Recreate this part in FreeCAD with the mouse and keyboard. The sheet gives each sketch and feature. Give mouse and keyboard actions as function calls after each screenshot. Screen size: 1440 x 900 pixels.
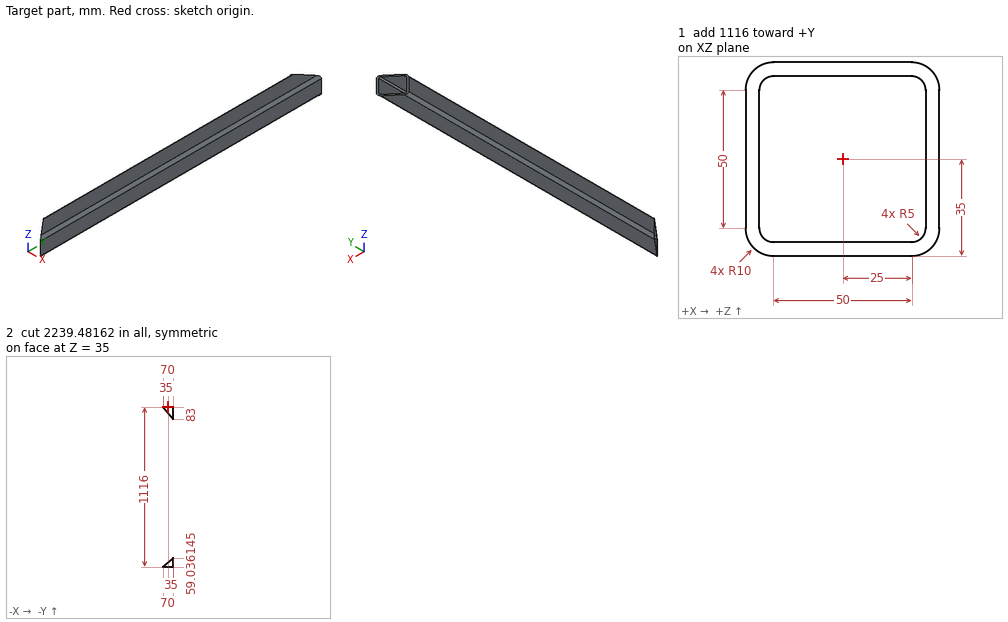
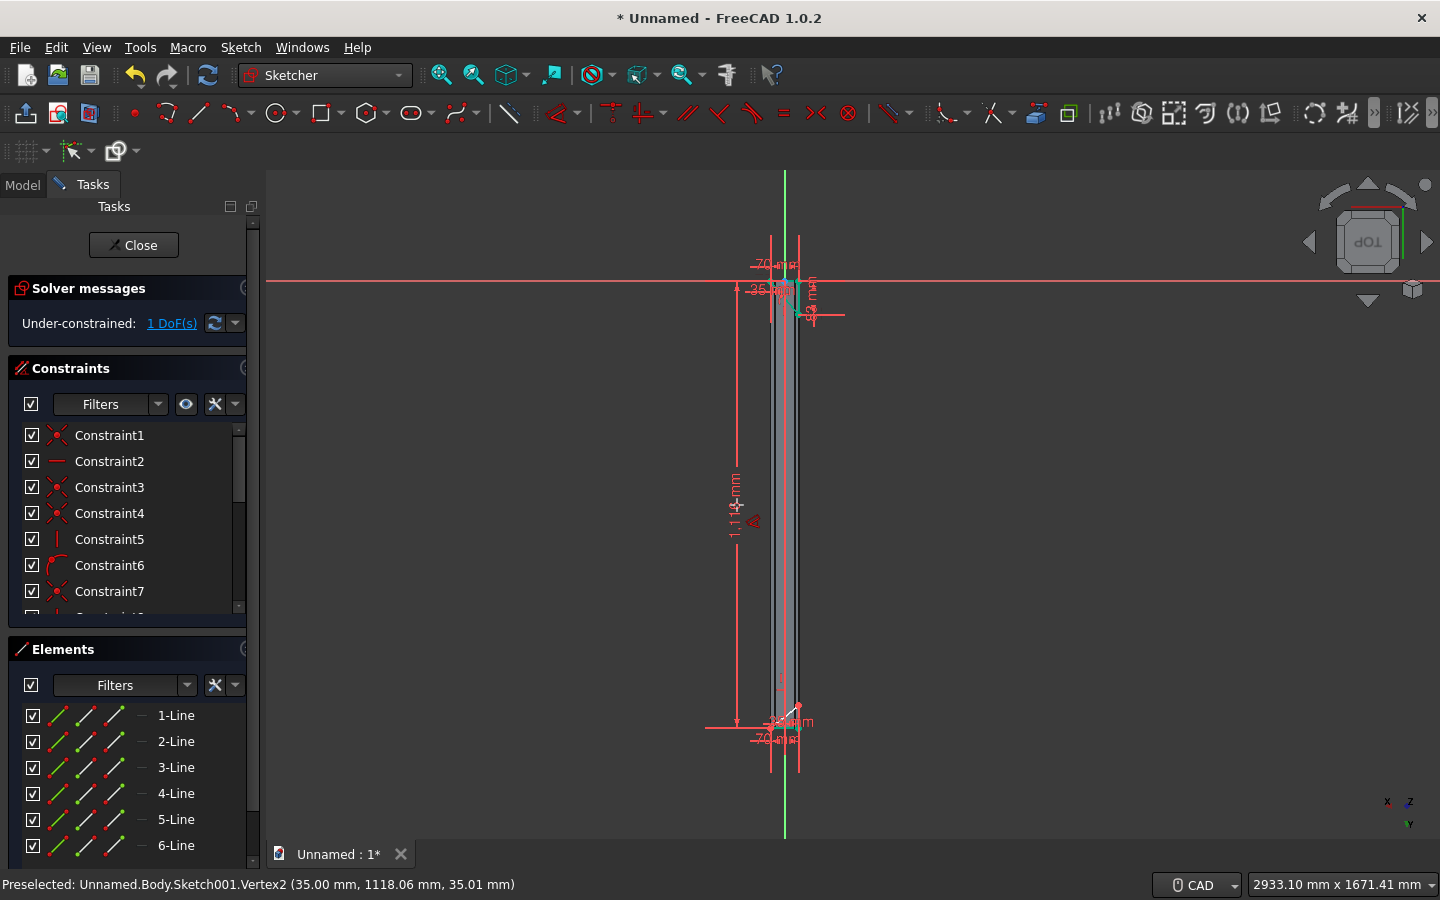
scroll(799, 719, up, 3)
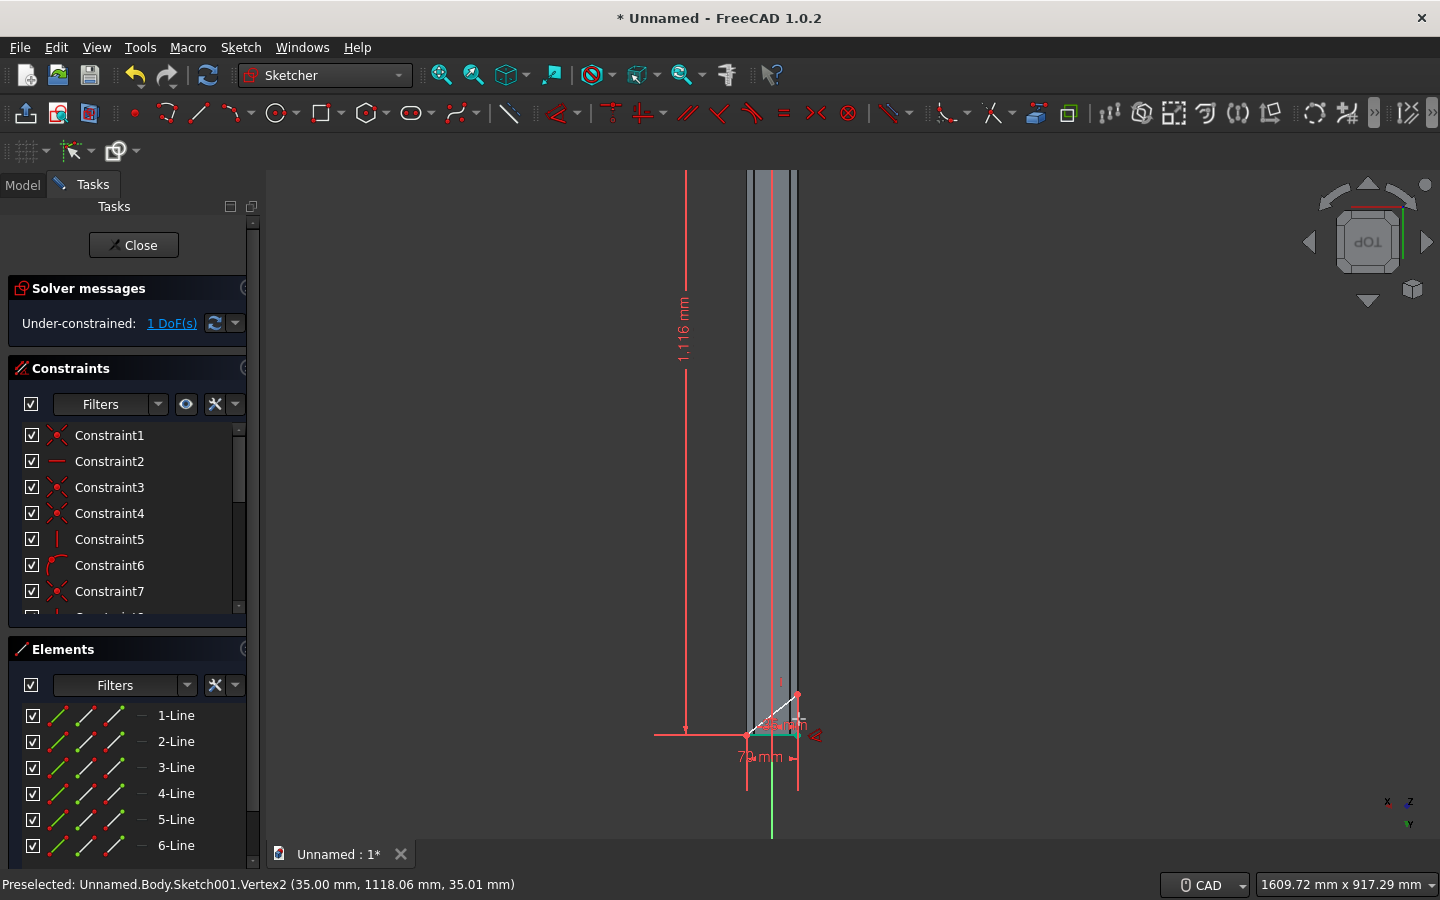
click(798, 719)
click(832, 706)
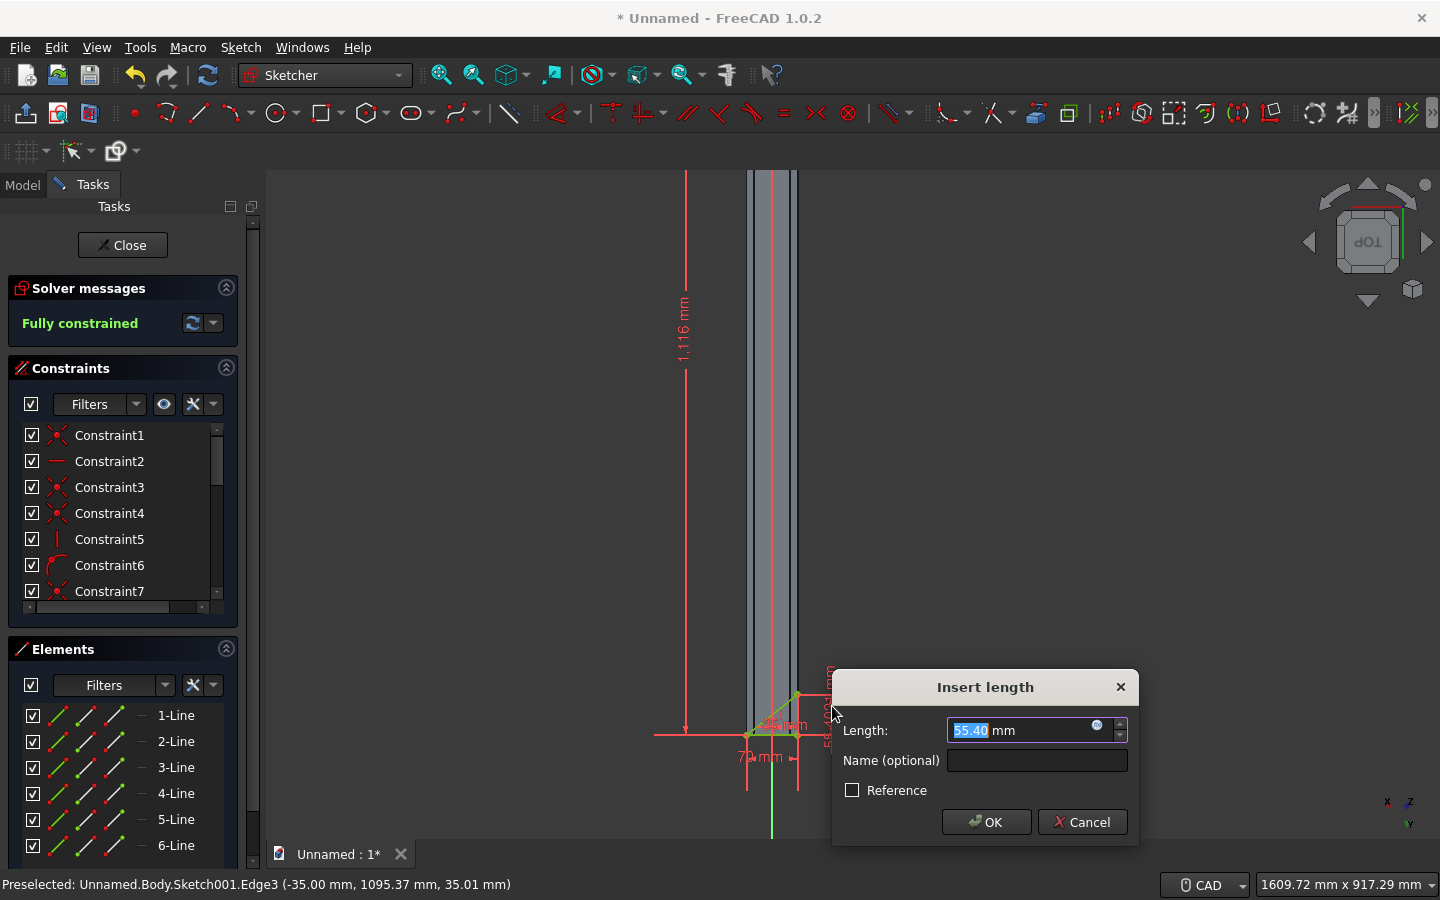
text(59.036145)
key(Return)
key(Escape)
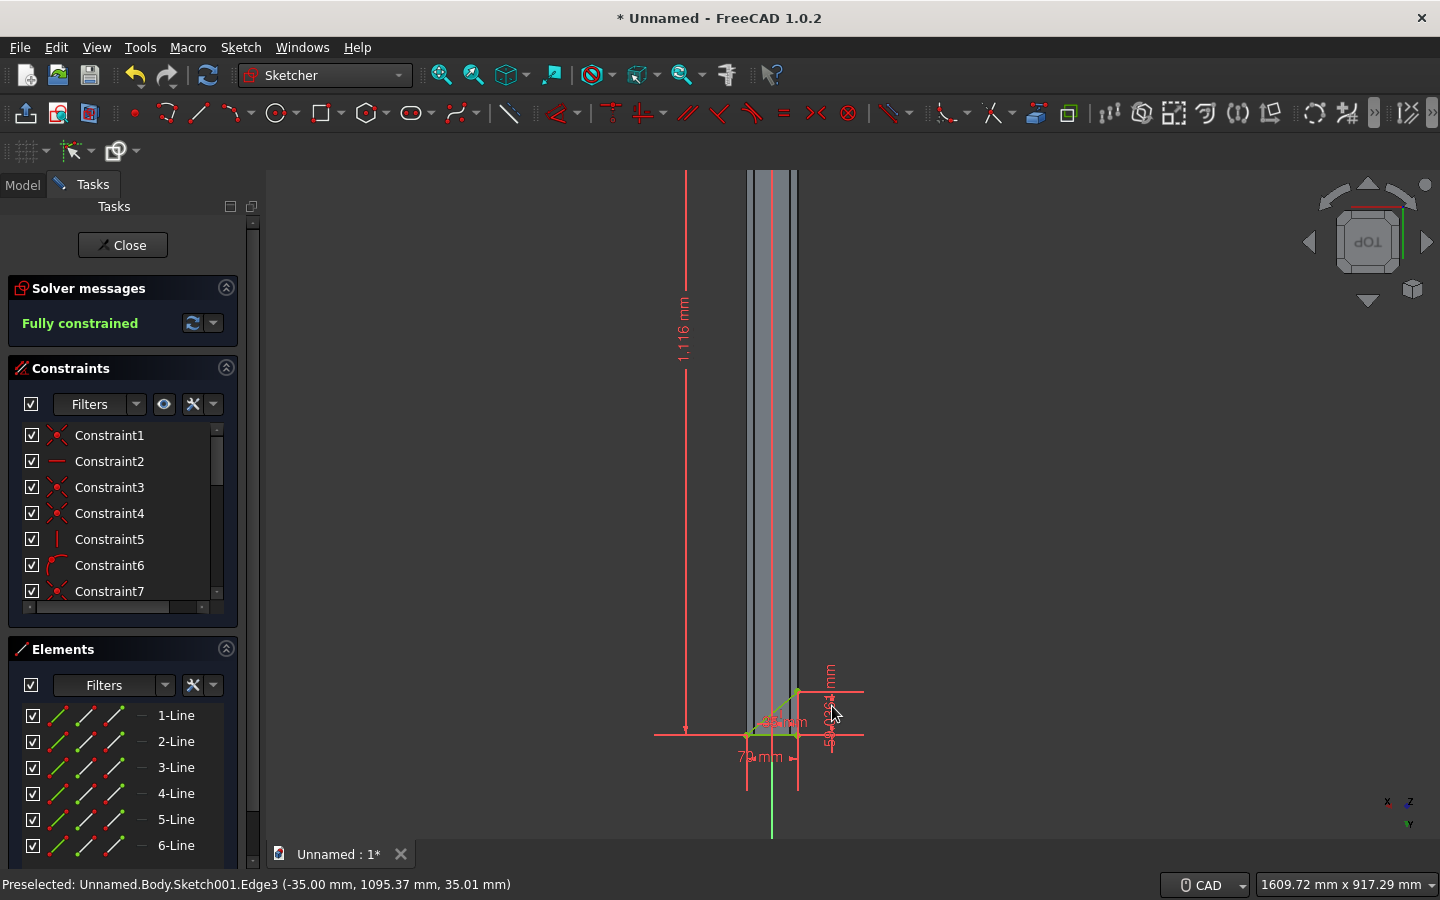
click(123, 245)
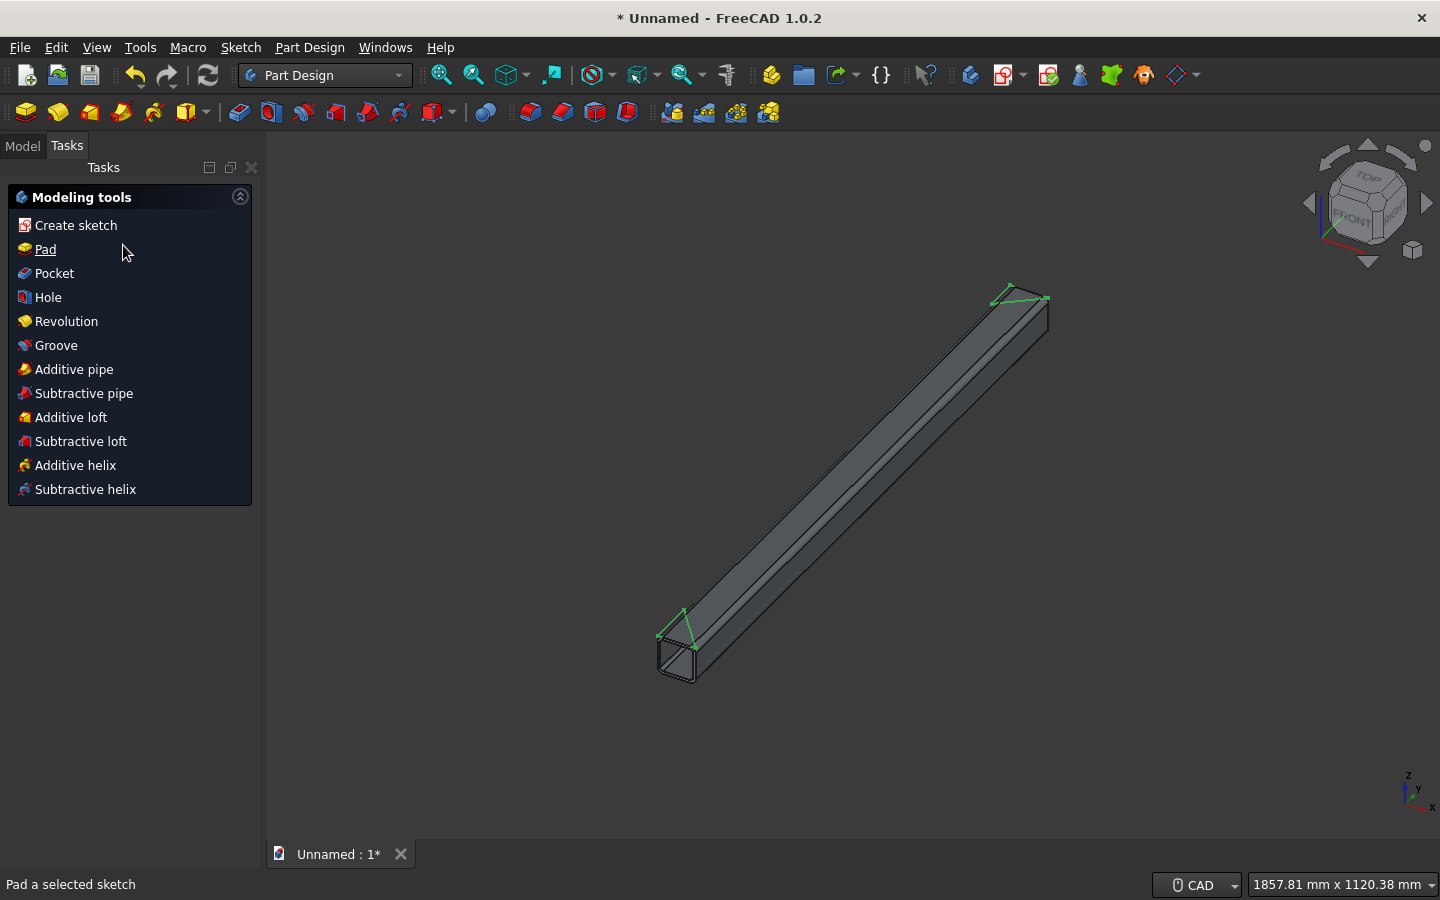
click(240, 112)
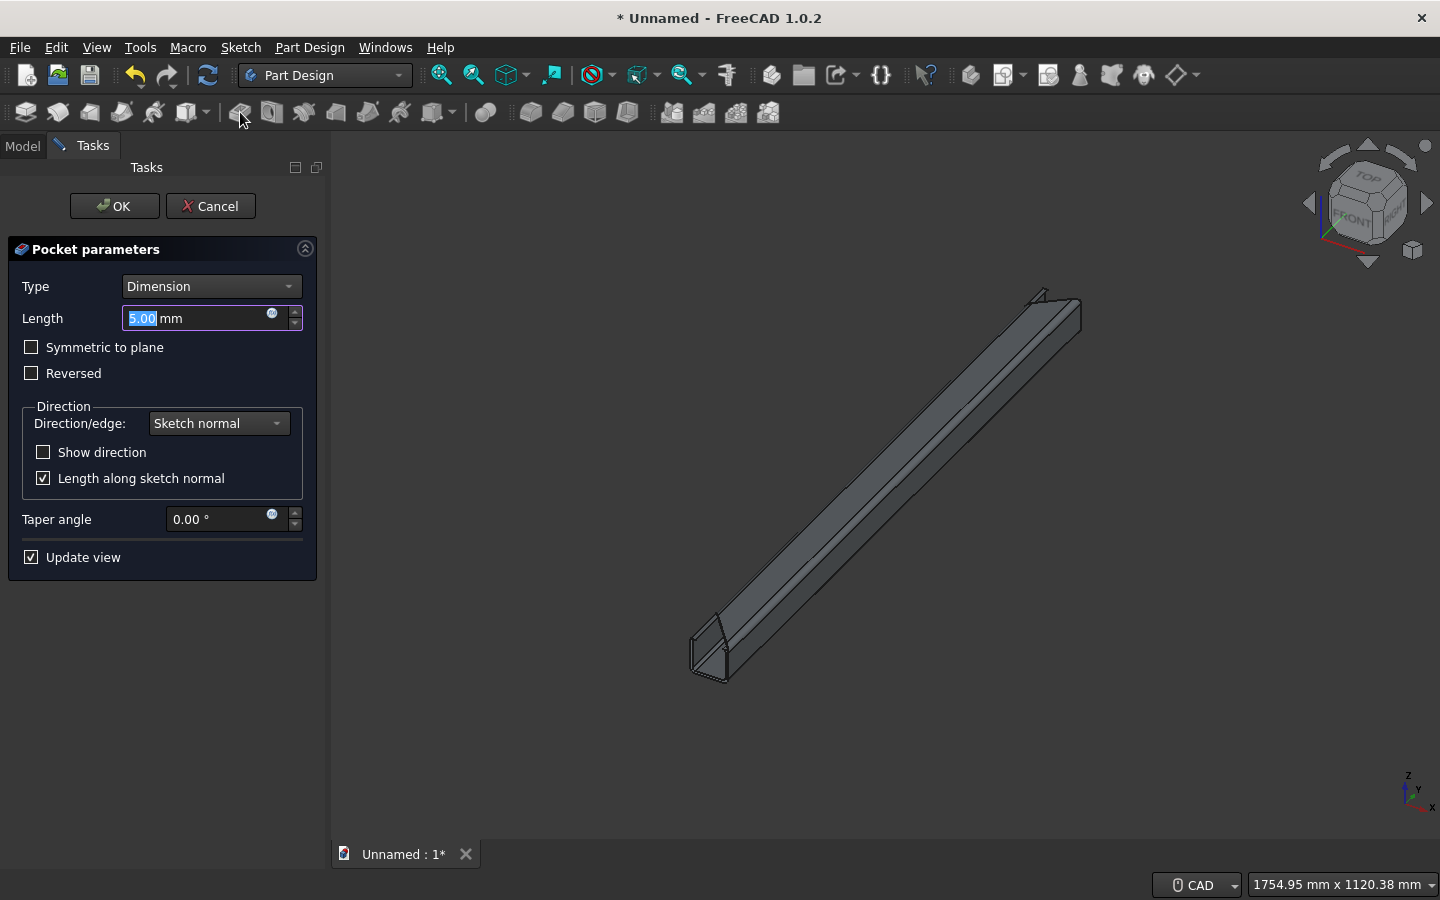
text(2239.48162)
key(Tab)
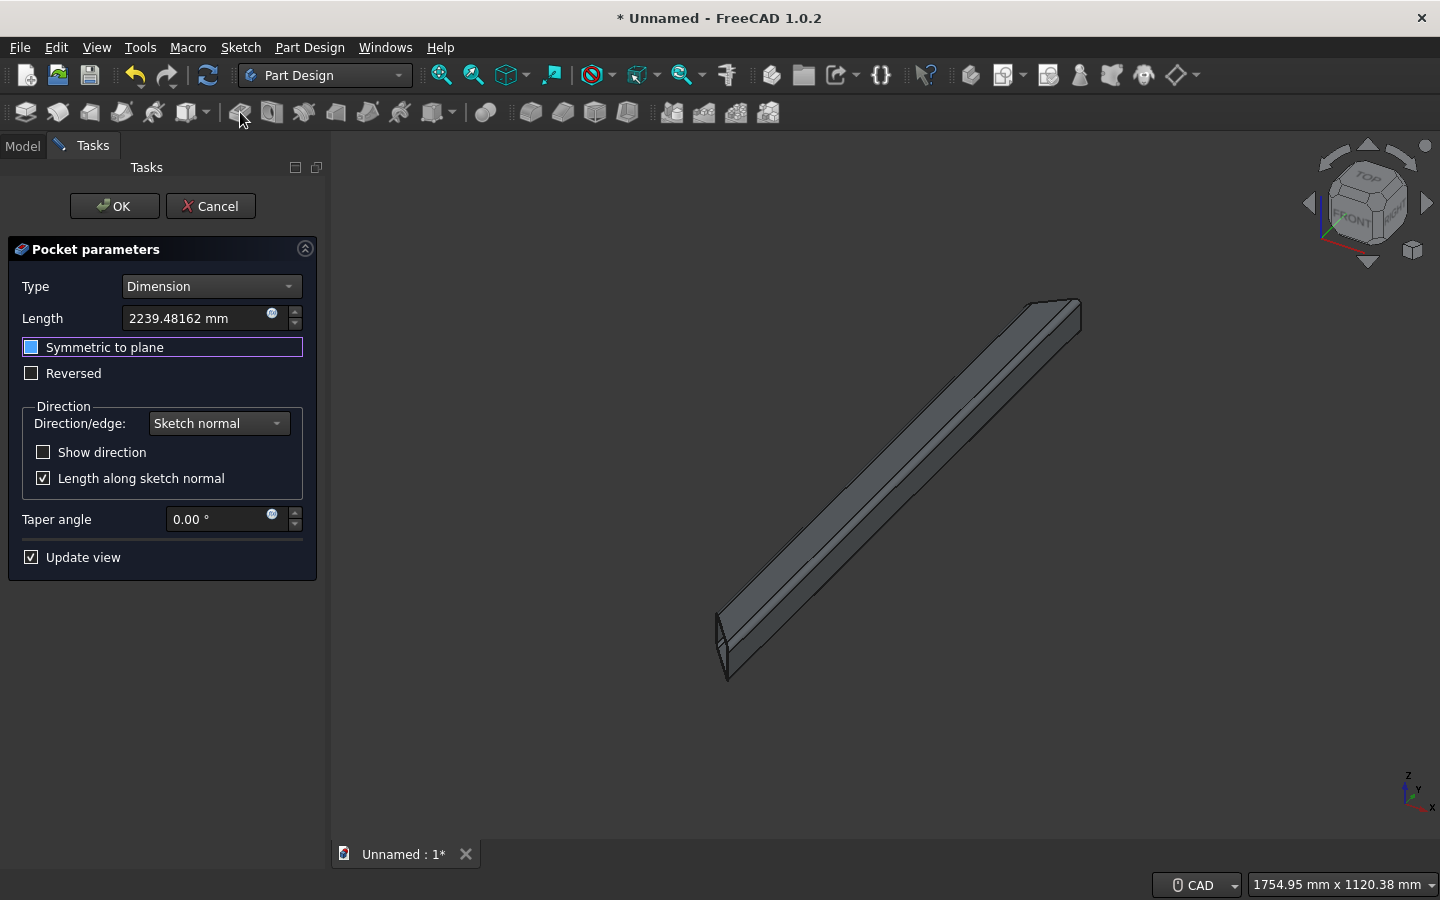
click(30, 347)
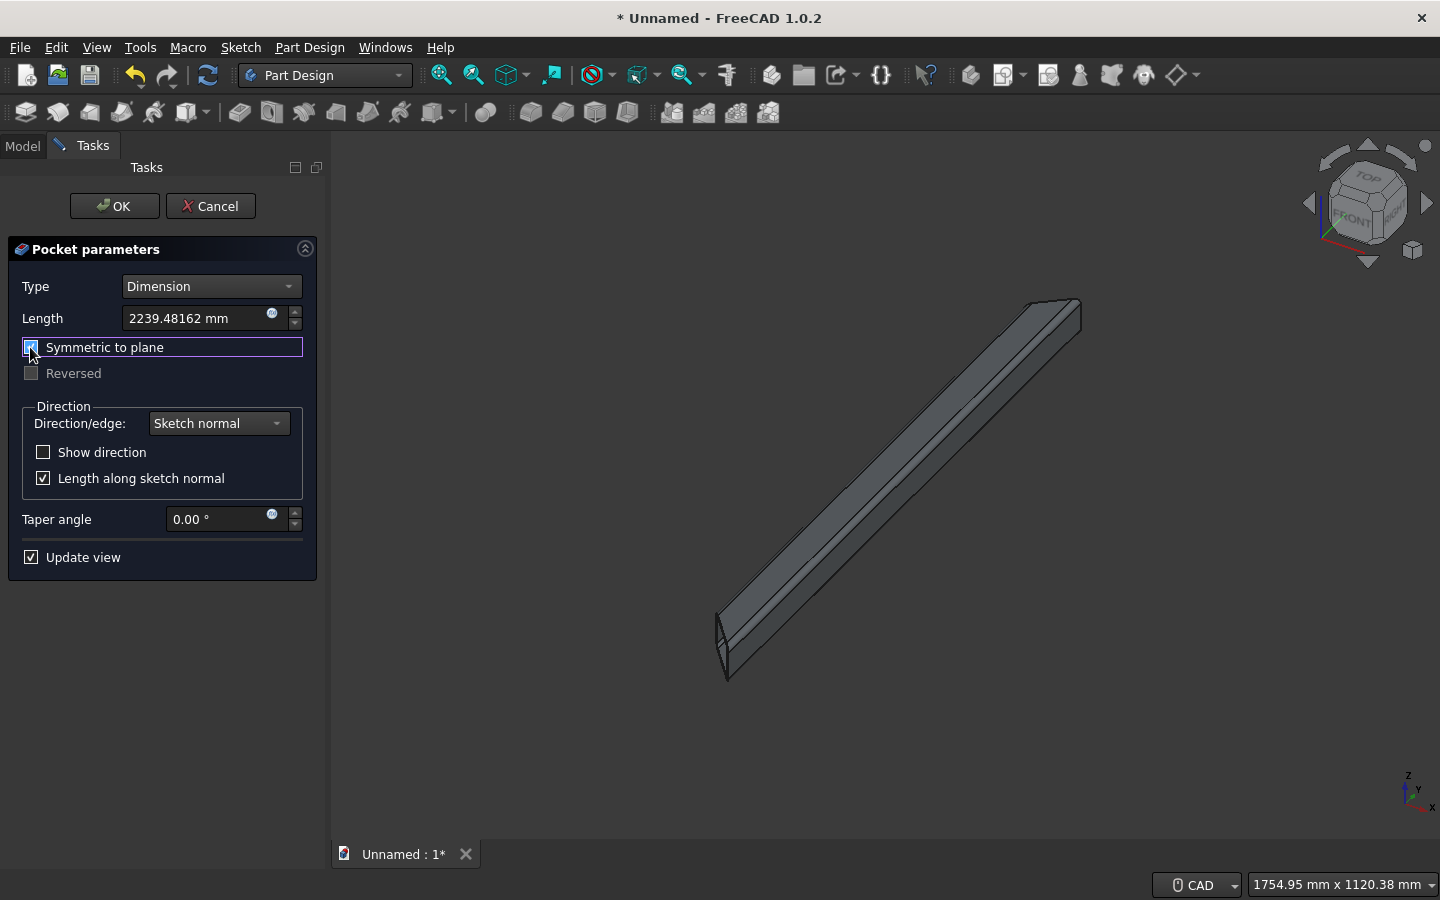
click(115, 206)